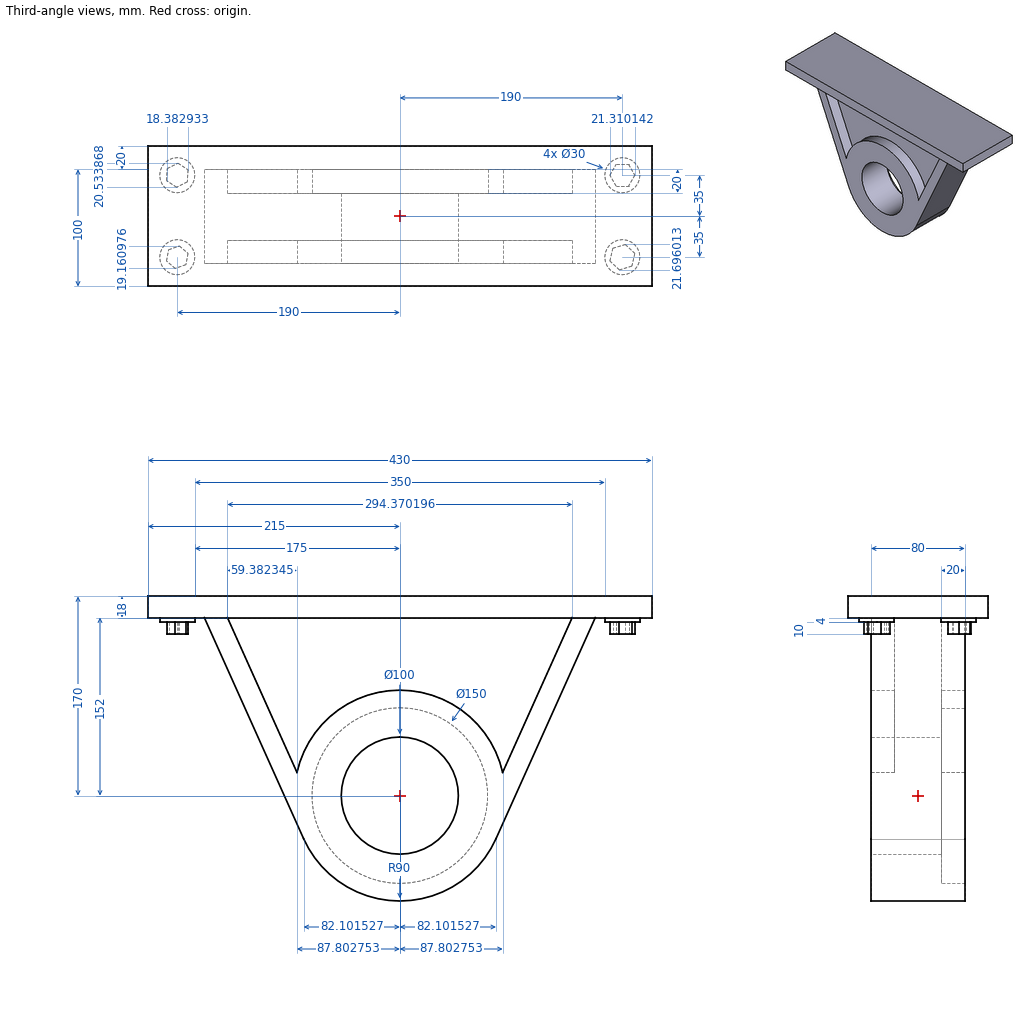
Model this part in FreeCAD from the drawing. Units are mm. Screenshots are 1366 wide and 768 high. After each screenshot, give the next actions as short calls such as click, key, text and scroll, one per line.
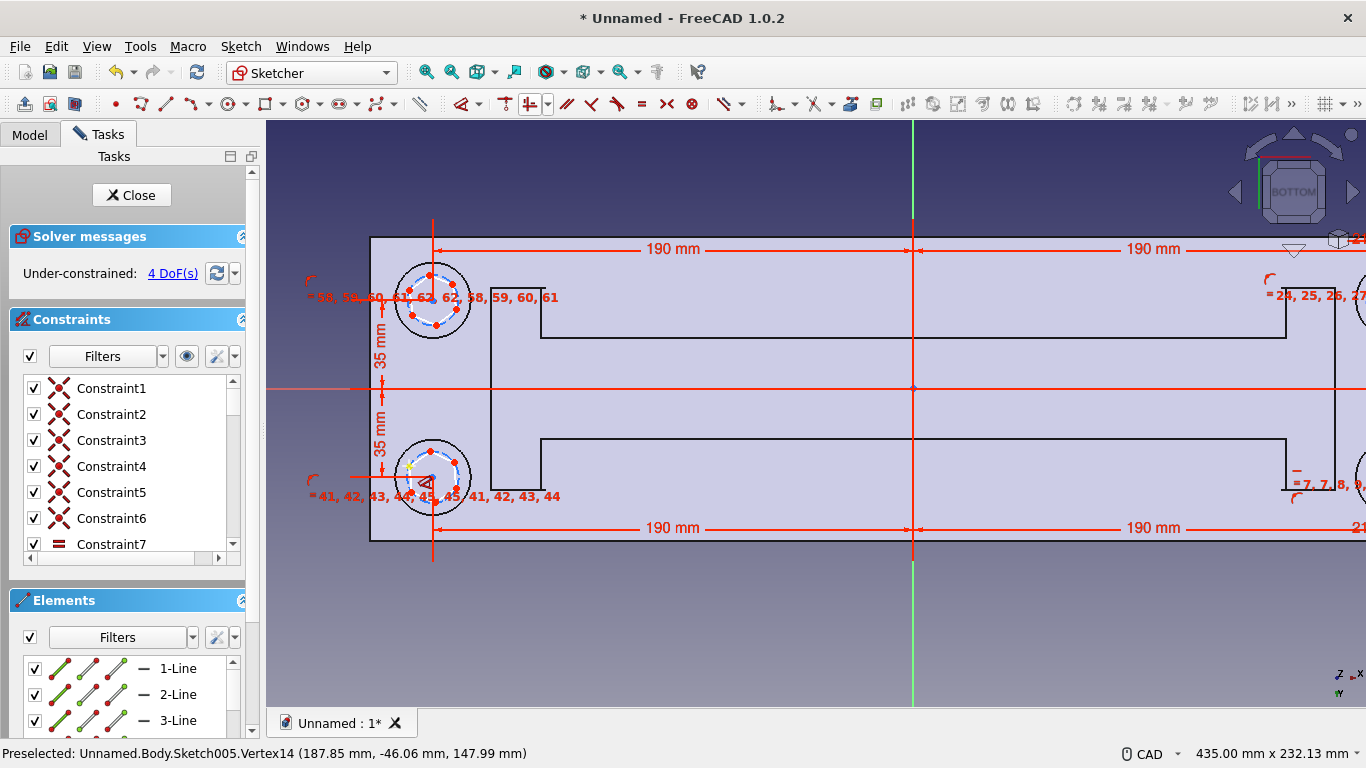
click(410, 466)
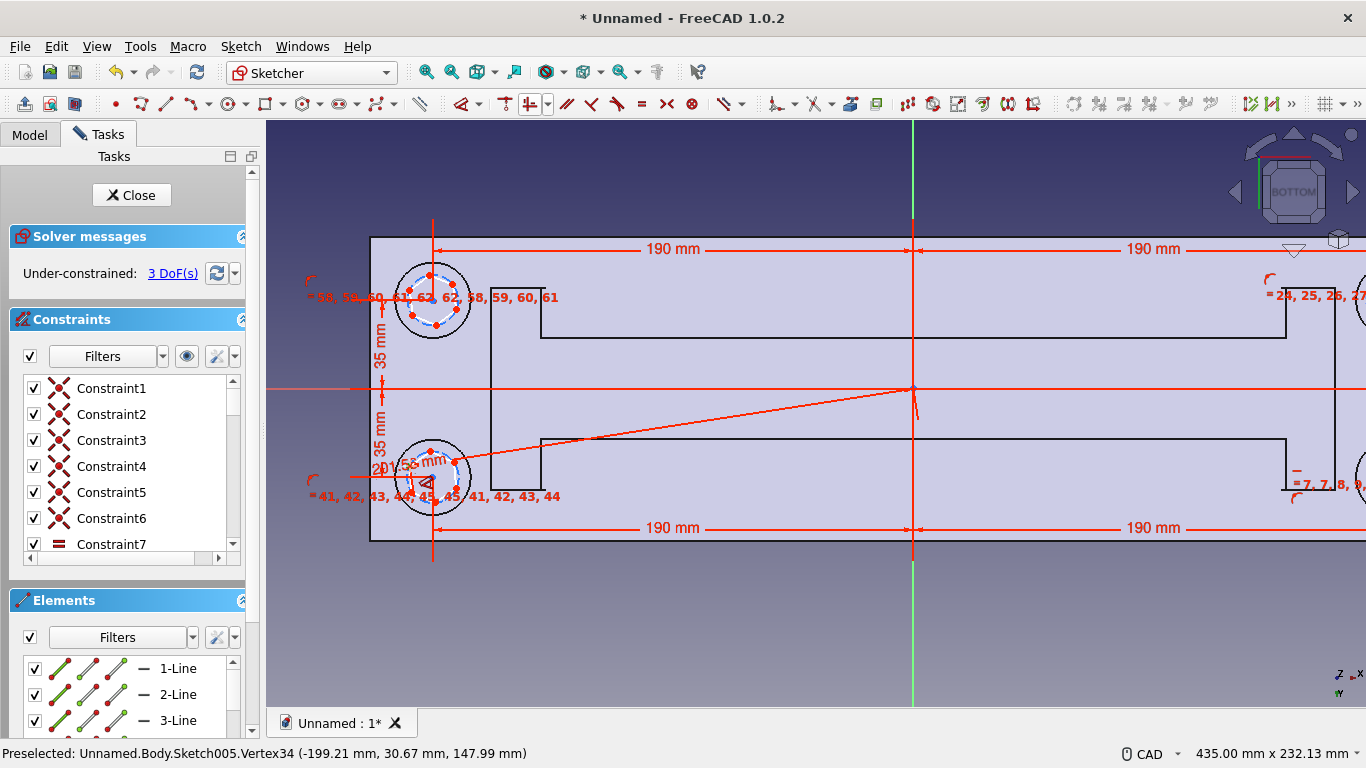
click(456, 488)
click(433, 522)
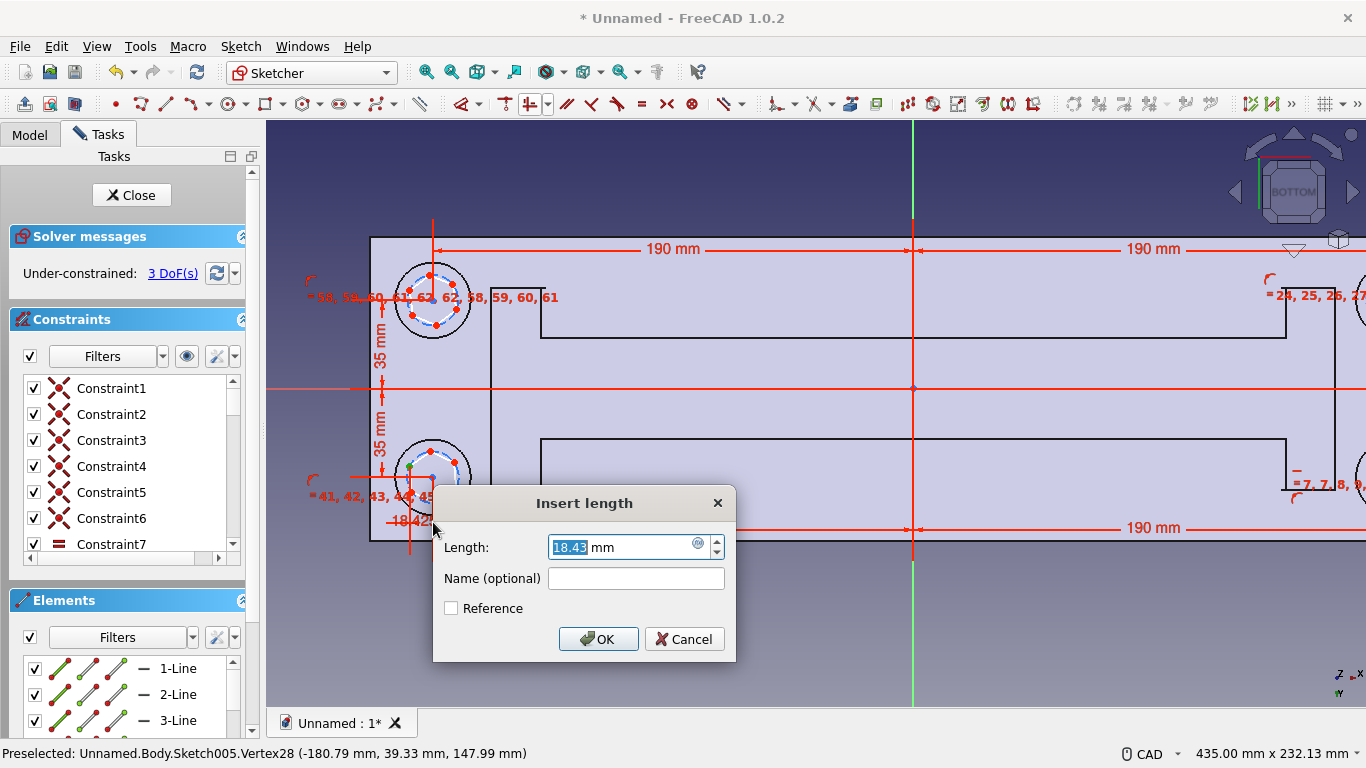
text(18.382933)
key(Return)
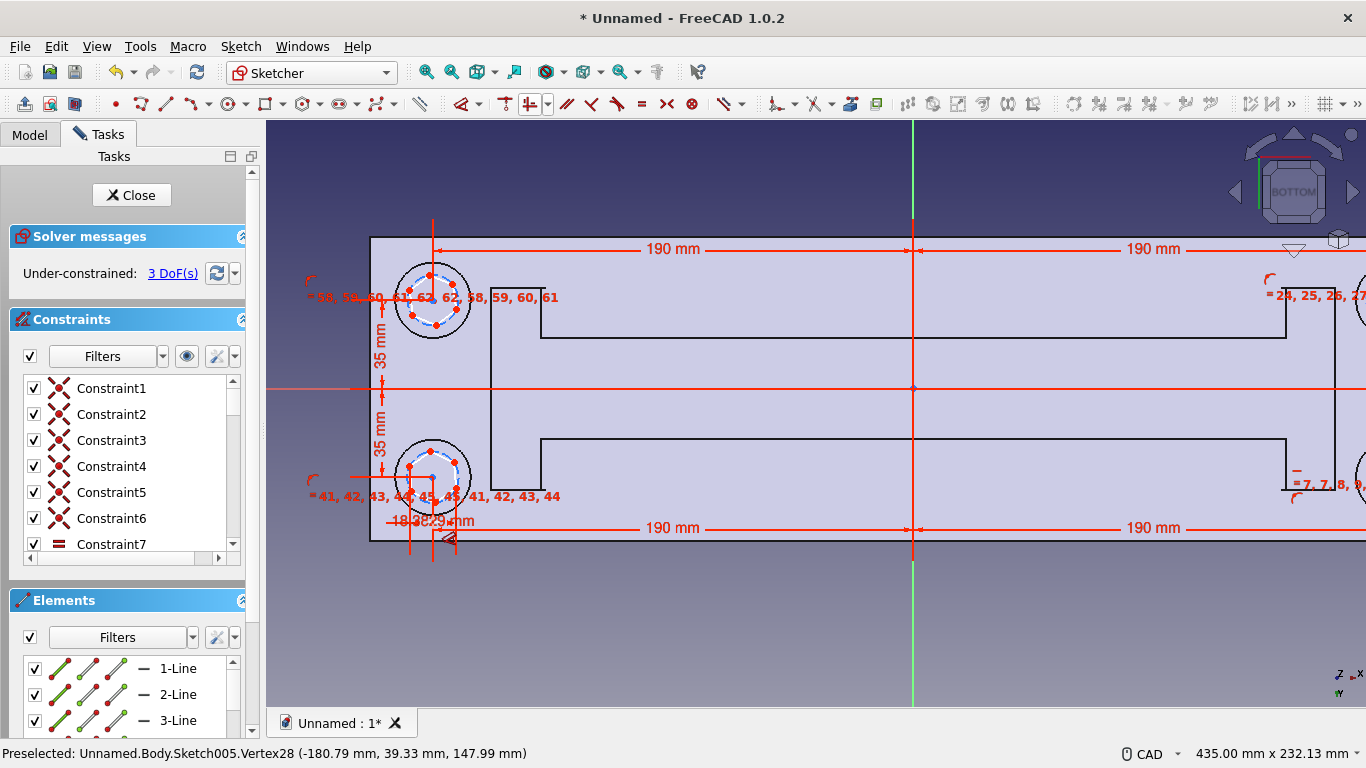
click(435, 503)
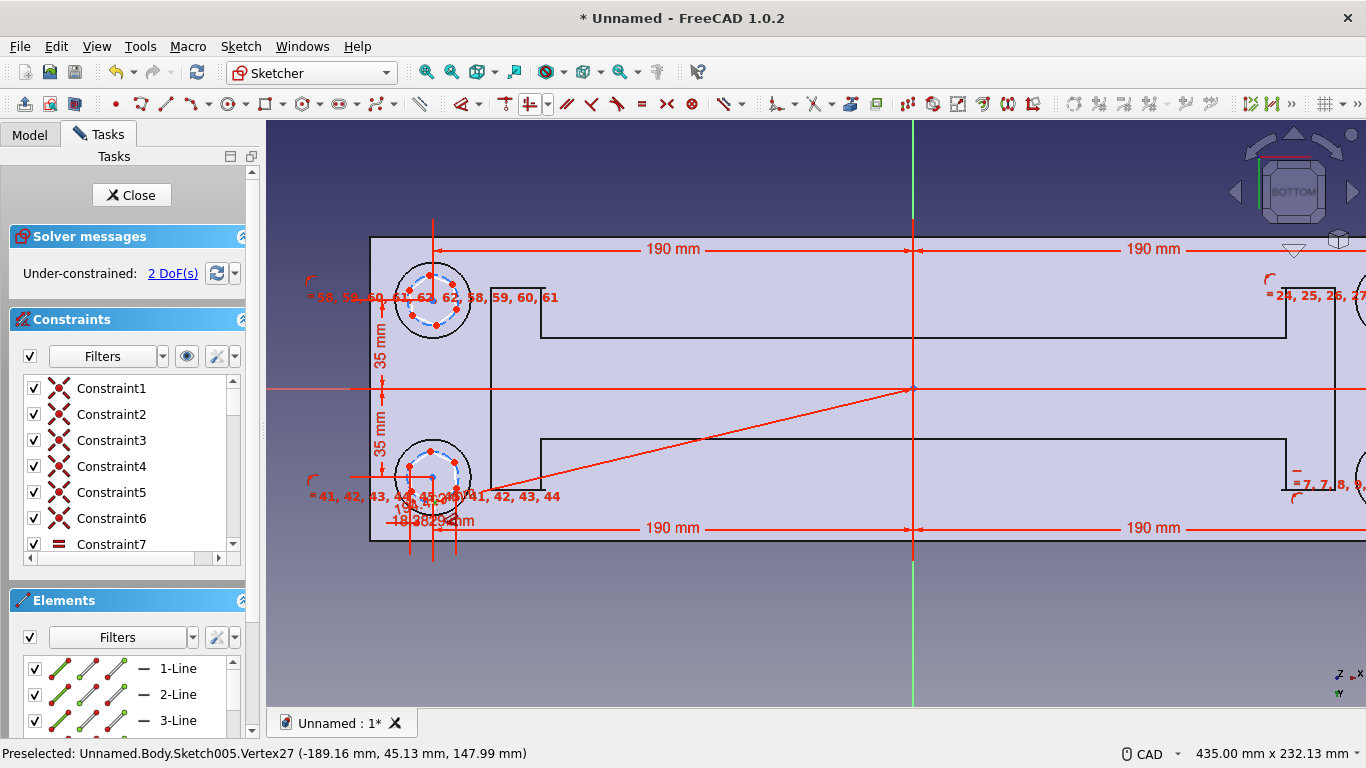
click(431, 452)
click(397, 459)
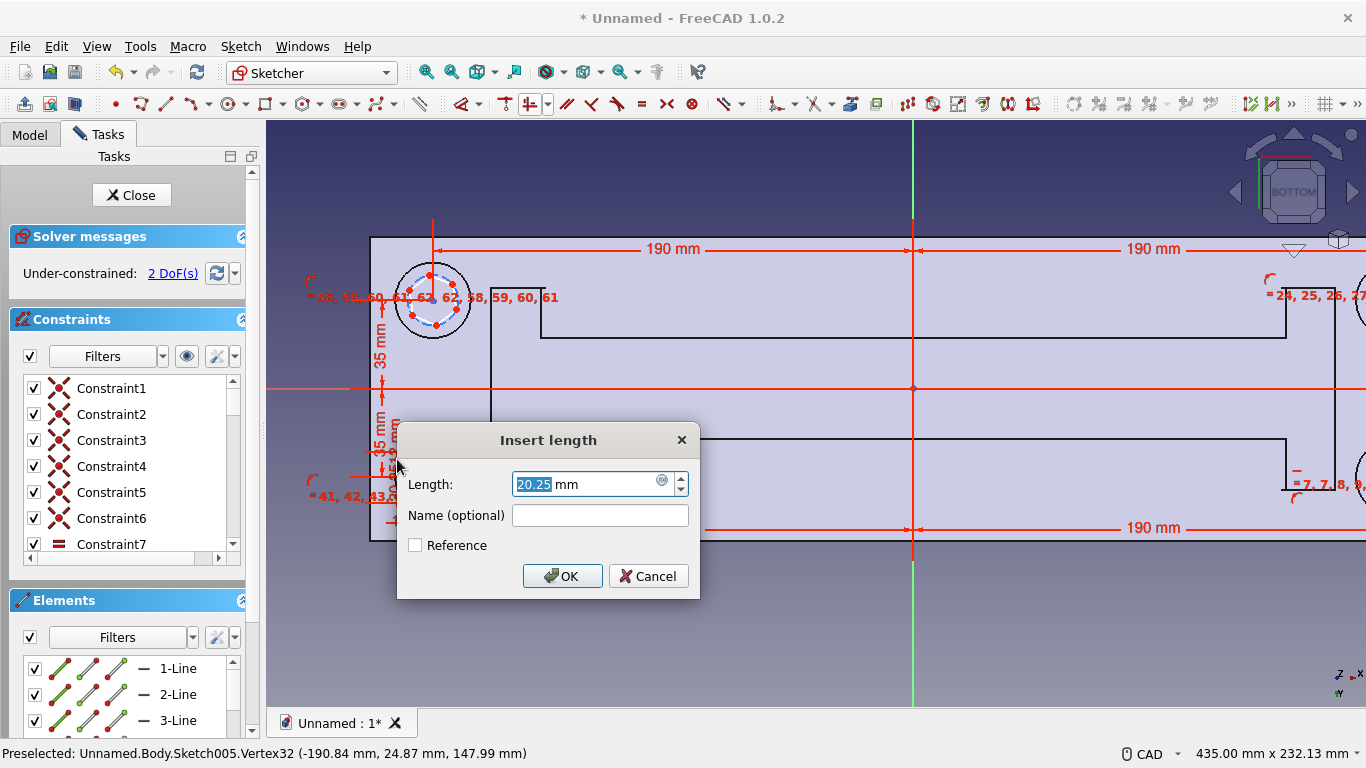
text(20.533868)
key(Return)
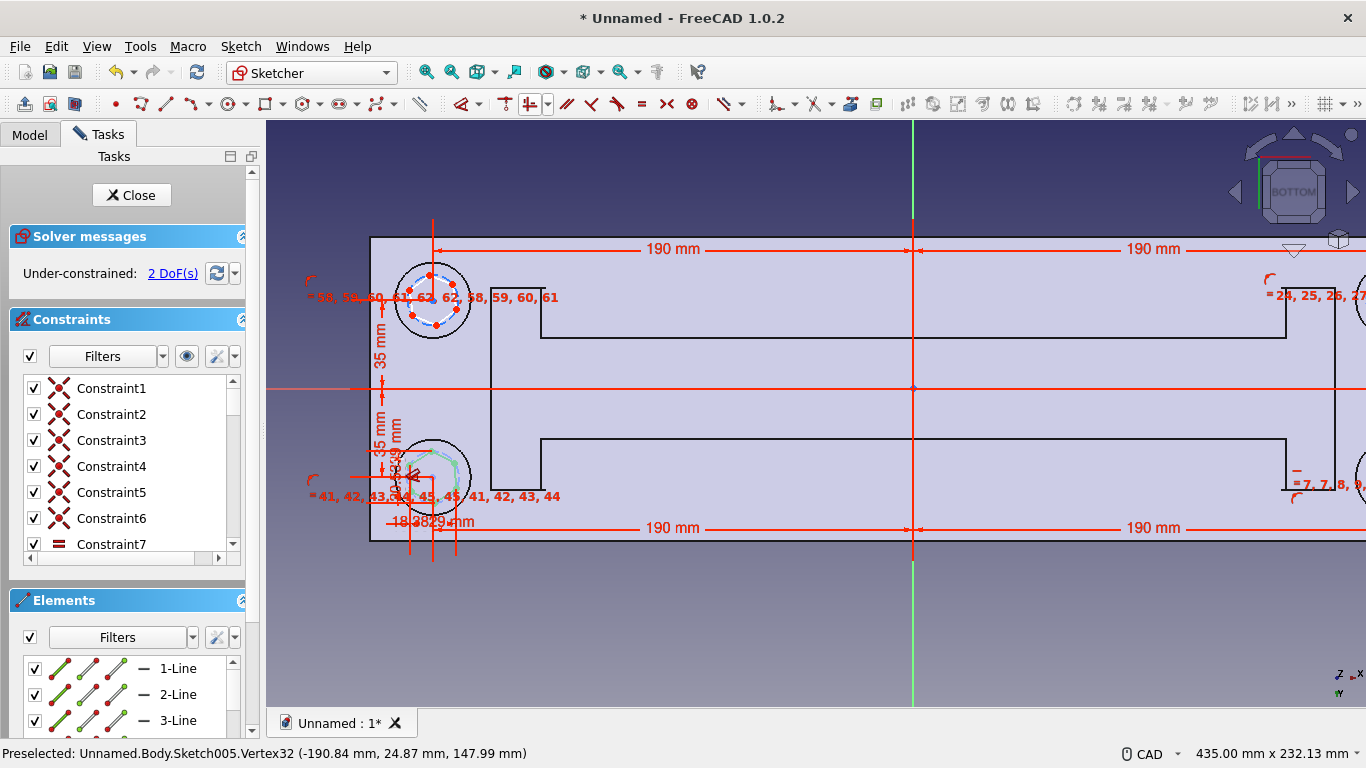
click(410, 291)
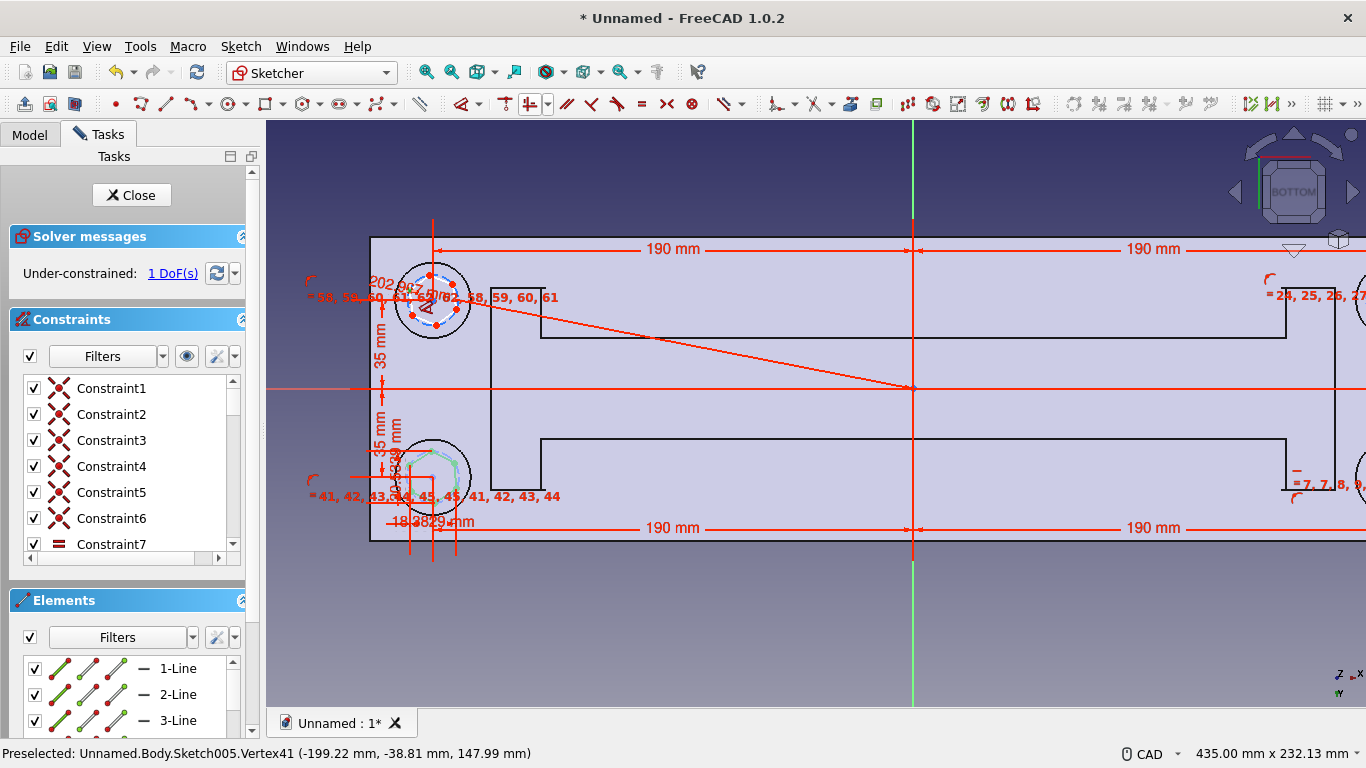
click(456, 310)
click(433, 257)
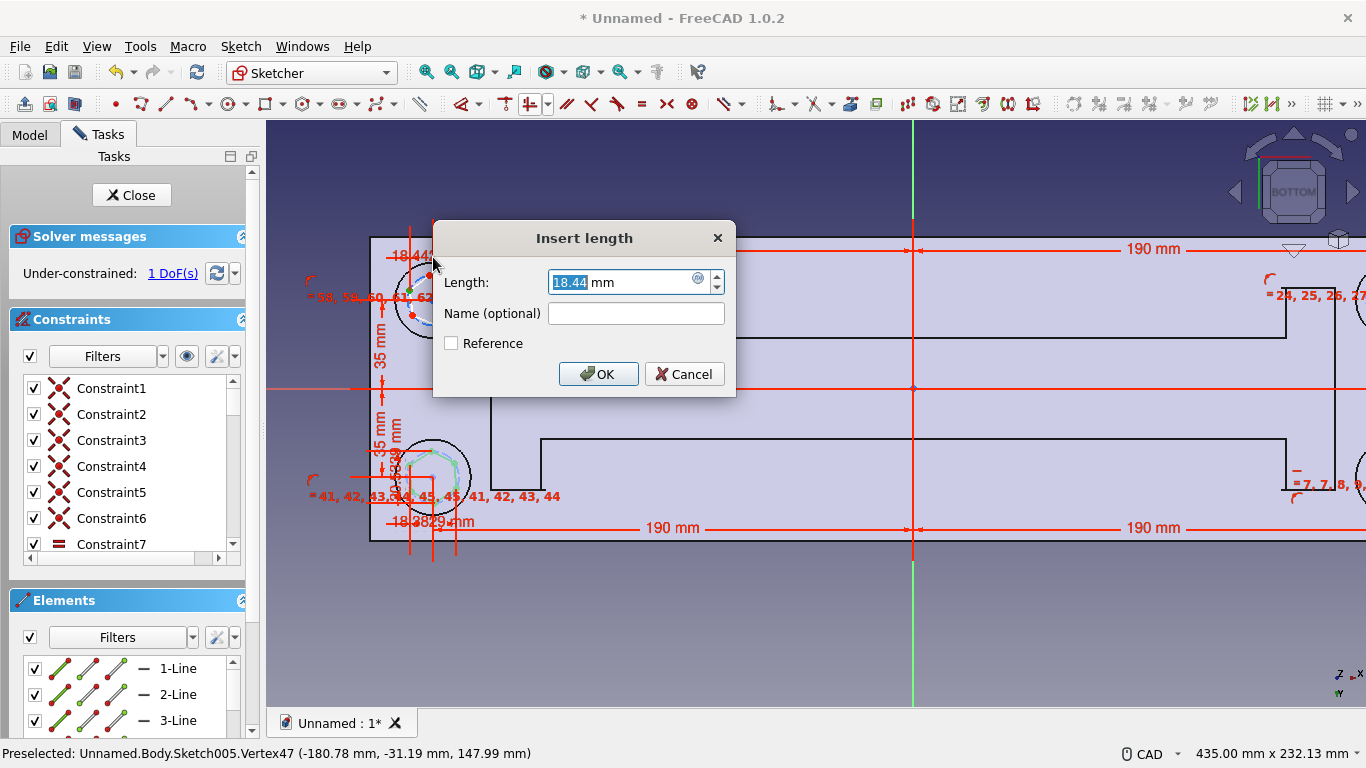
text(18.382933)
key(Return)